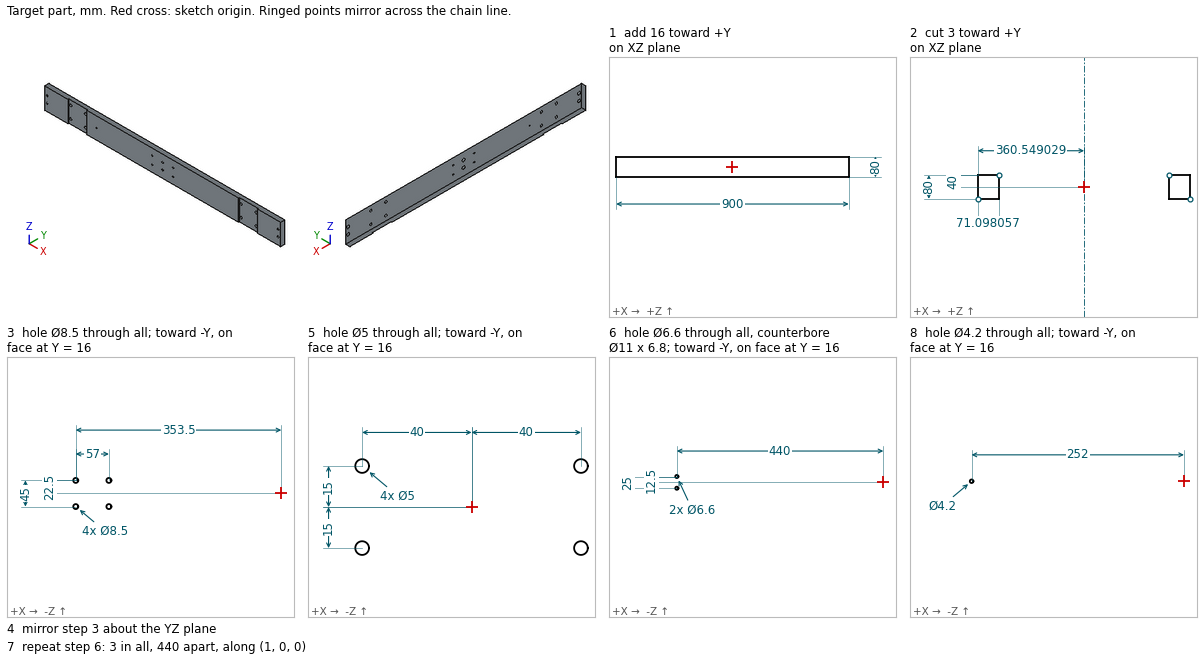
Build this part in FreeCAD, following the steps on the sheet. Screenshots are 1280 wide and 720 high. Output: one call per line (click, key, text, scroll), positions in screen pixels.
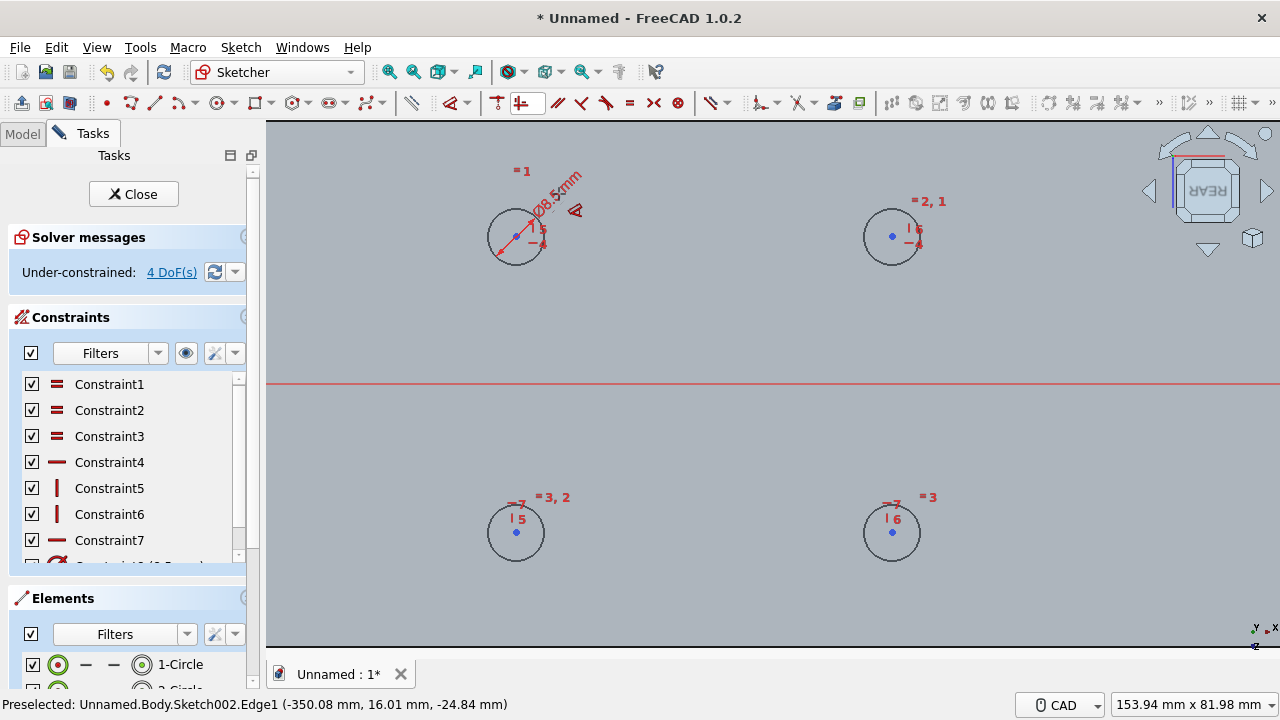
click(516, 237)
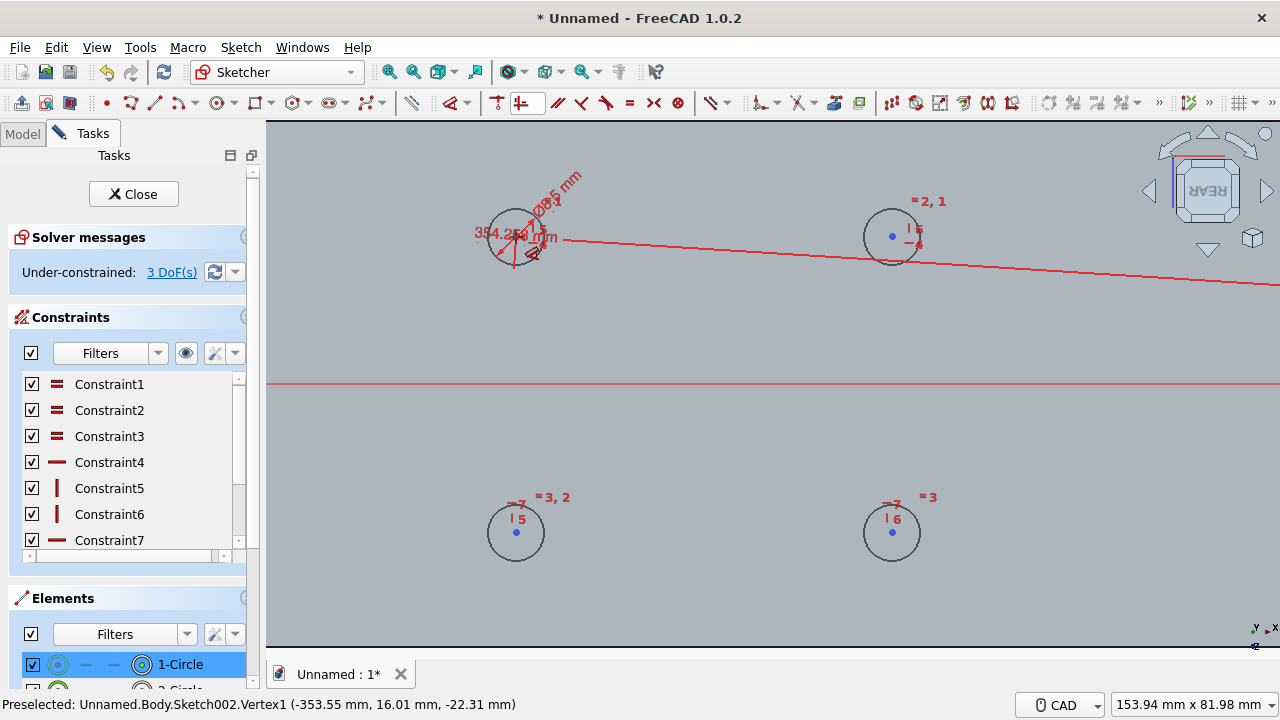
click(892, 237)
click(704, 203)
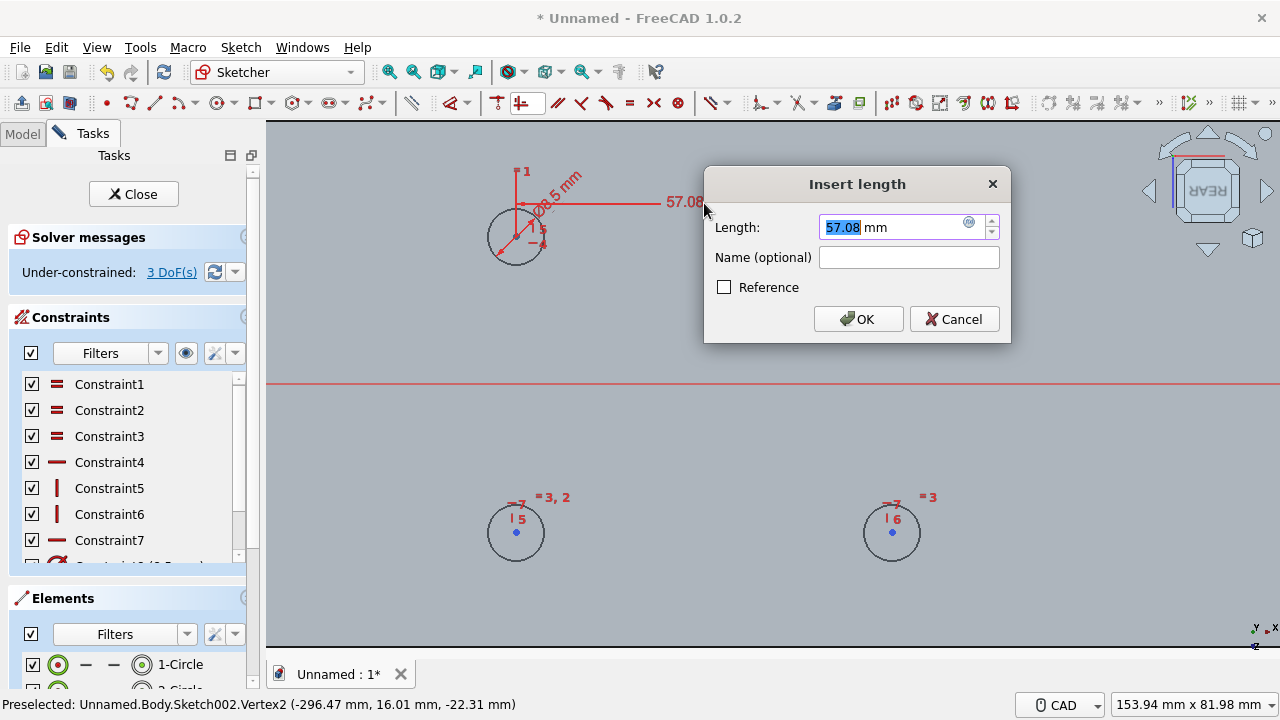
text(57)
key(Return)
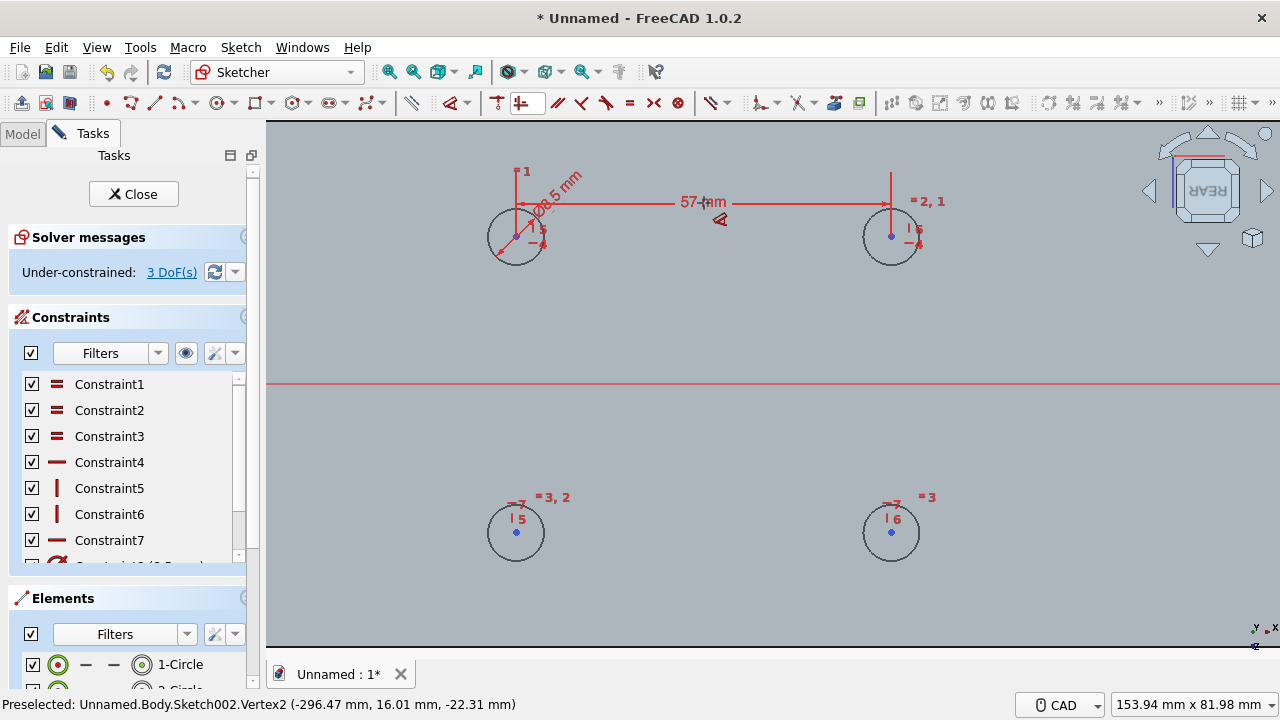
click(516, 237)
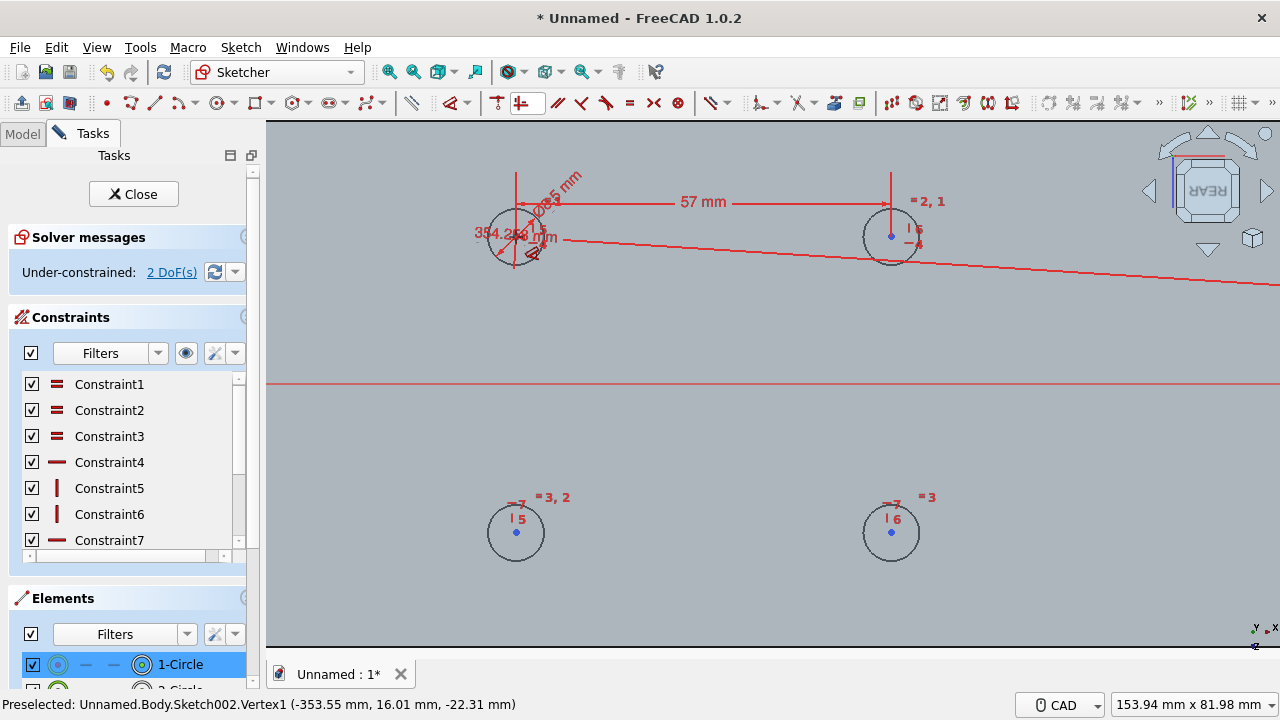
click(516, 533)
click(482, 317)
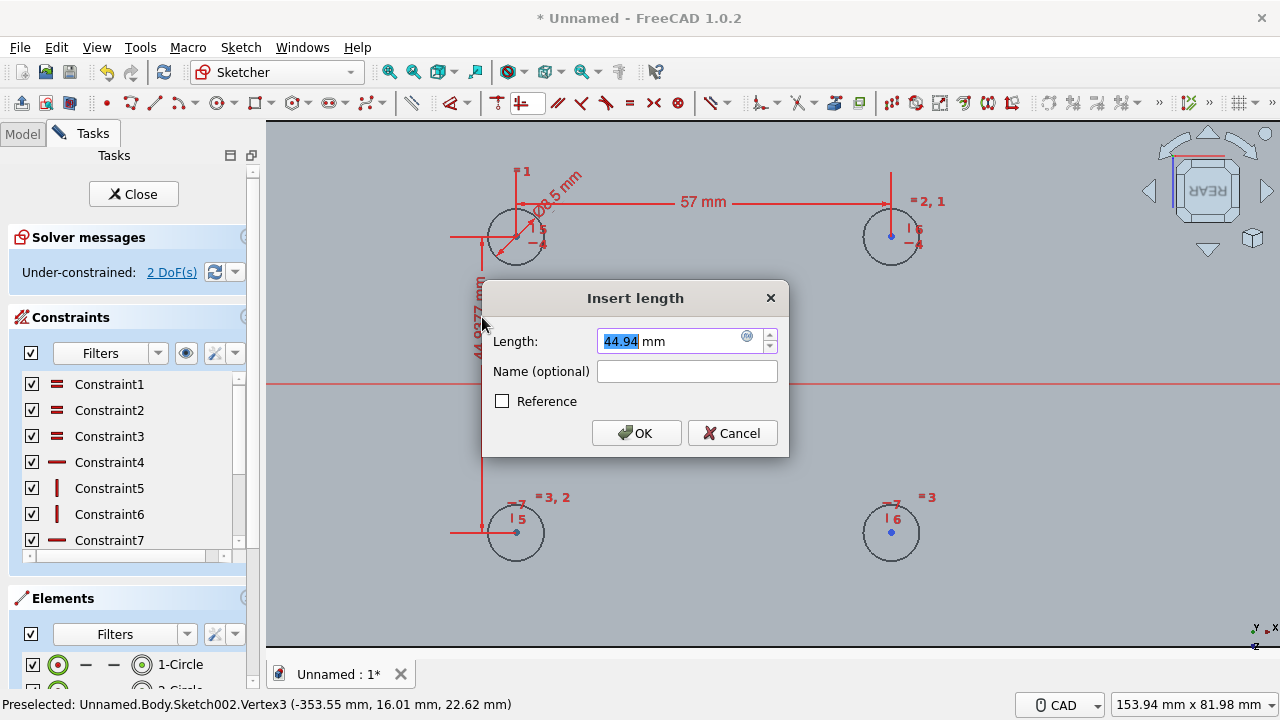
text(45)
key(Return)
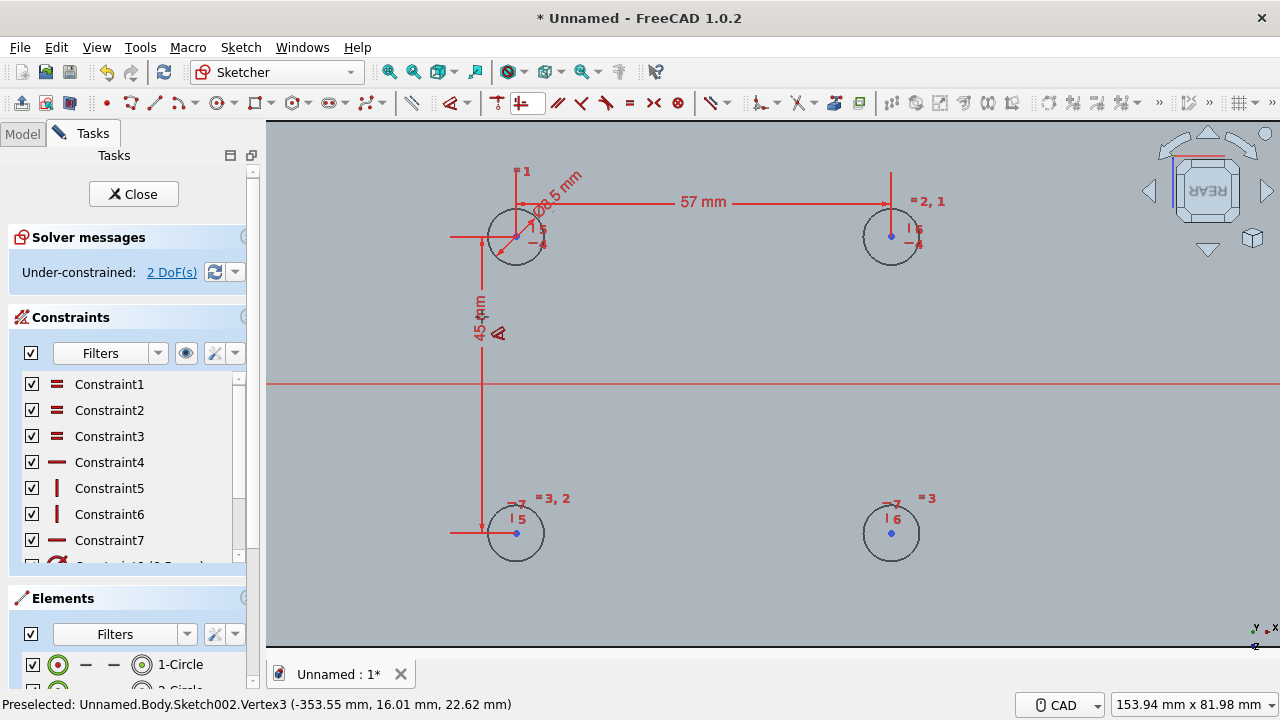
click(516, 237)
click(482, 277)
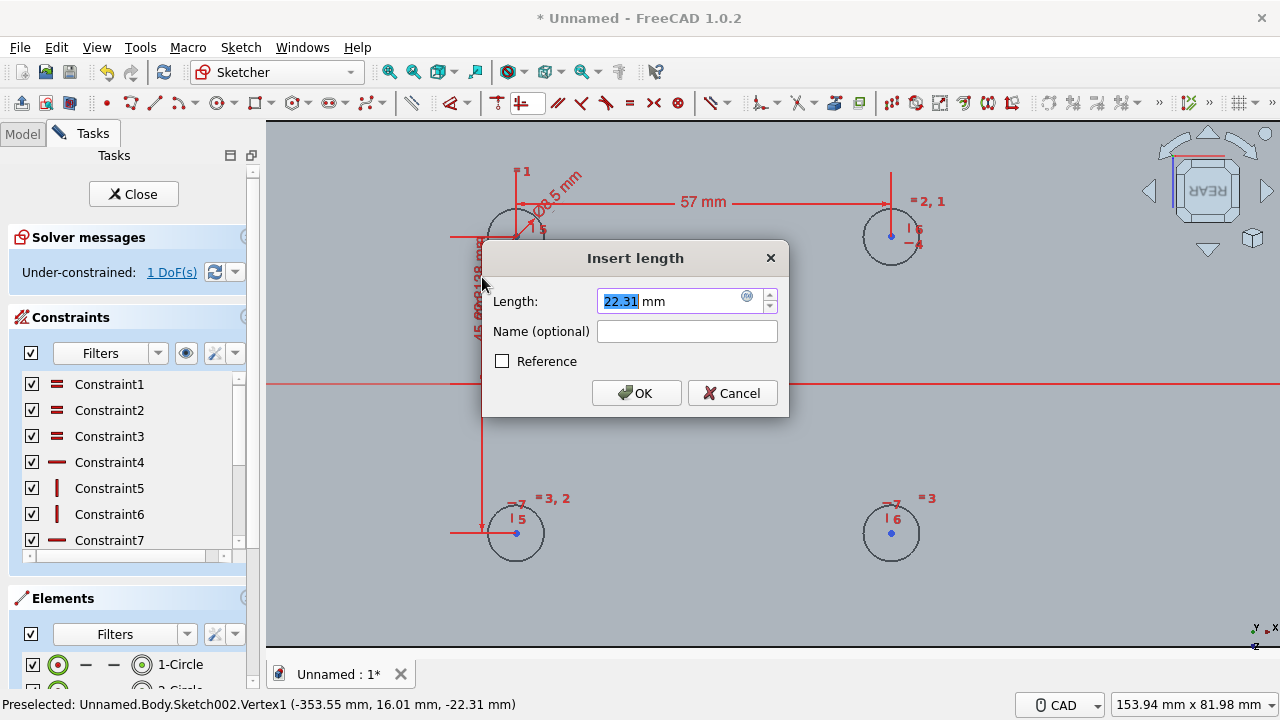
text(22.5)
key(Return)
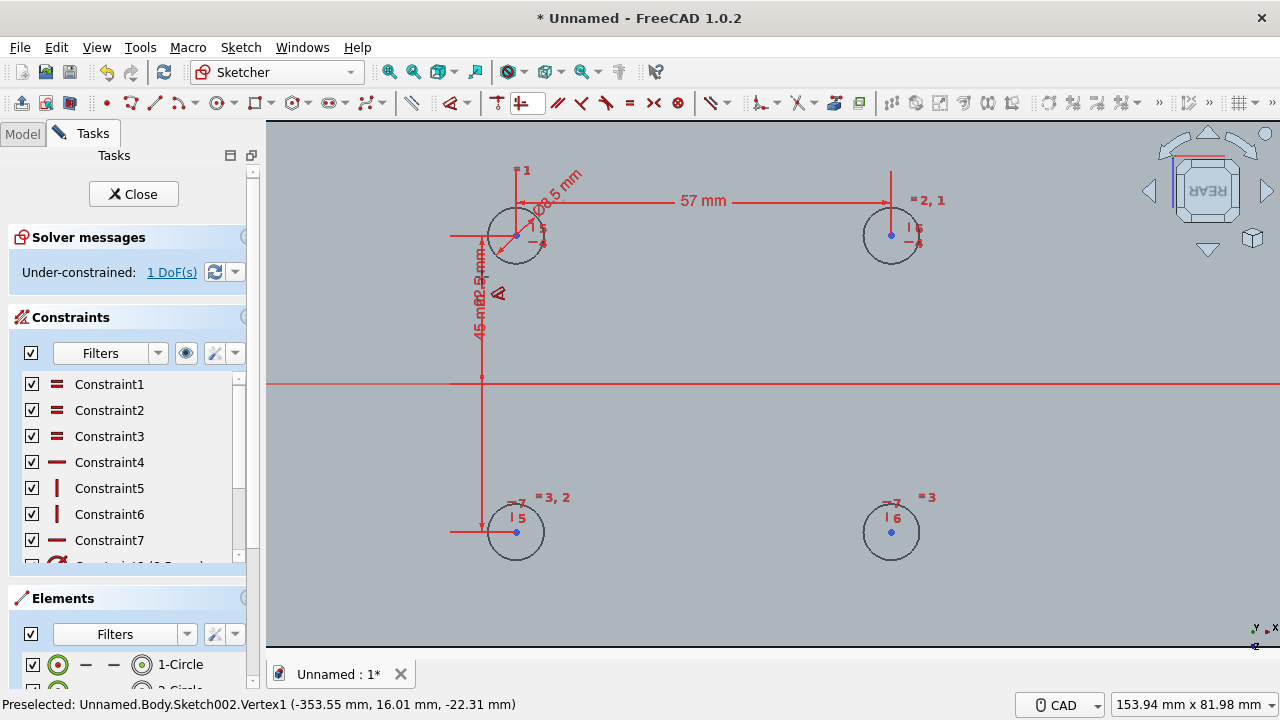
click(516, 236)
click(816, 202)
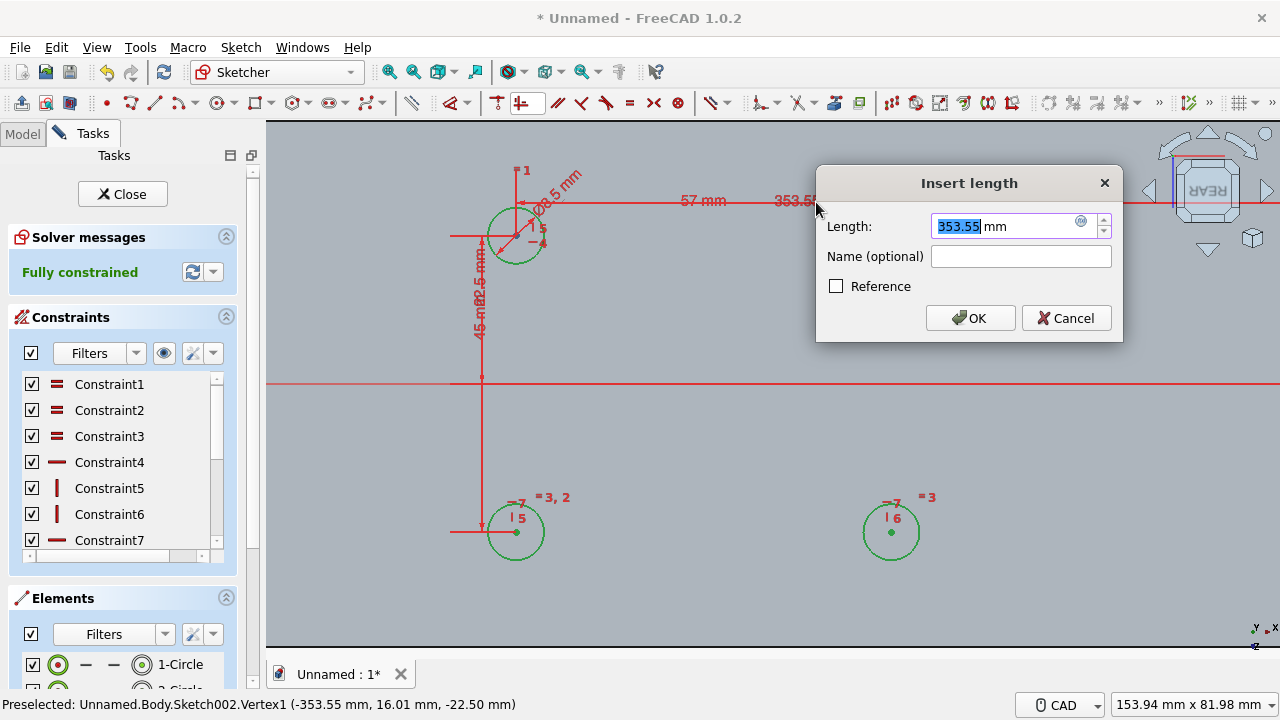
text(353.5)
key(Return)
key(Escape)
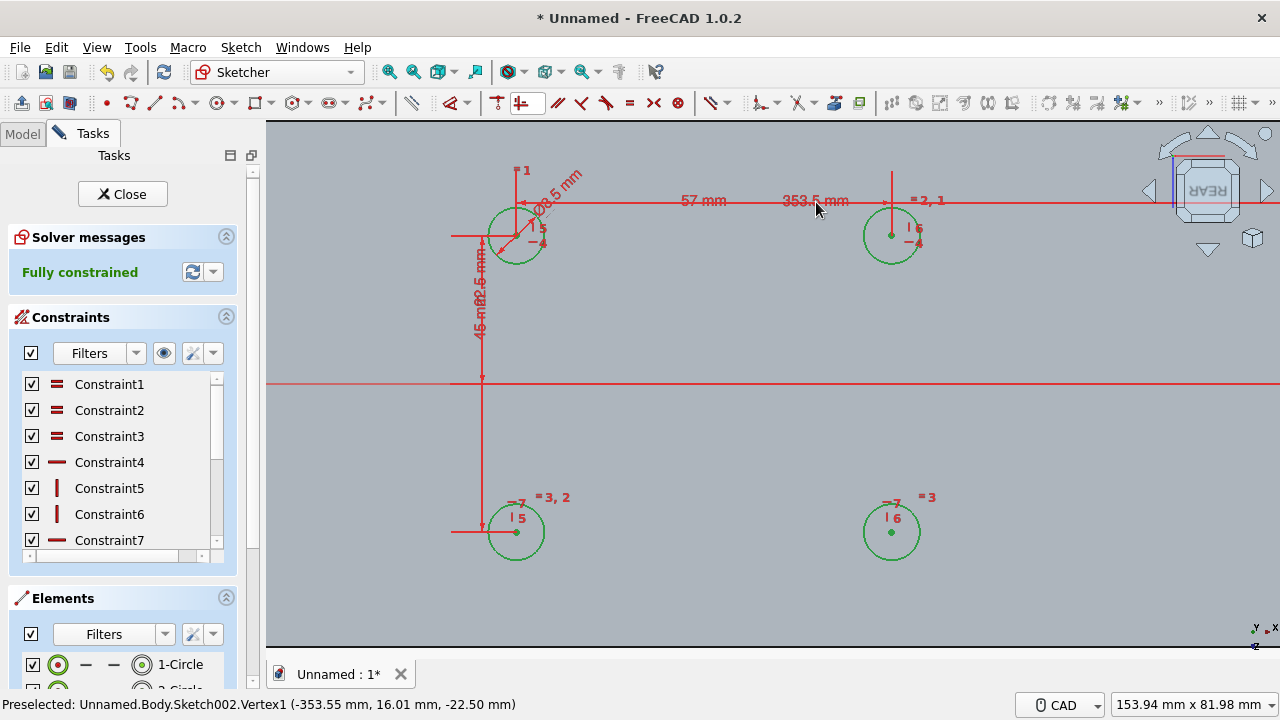
click(123, 194)